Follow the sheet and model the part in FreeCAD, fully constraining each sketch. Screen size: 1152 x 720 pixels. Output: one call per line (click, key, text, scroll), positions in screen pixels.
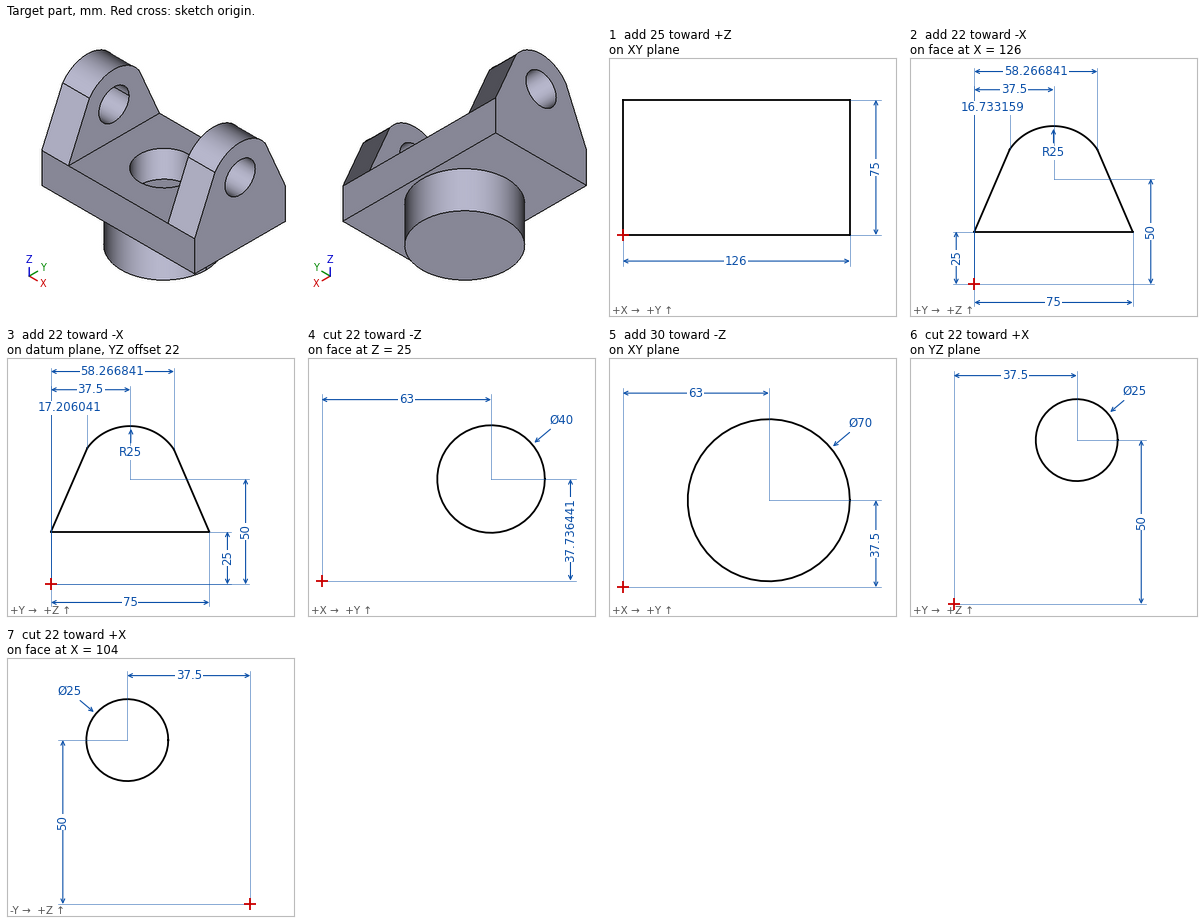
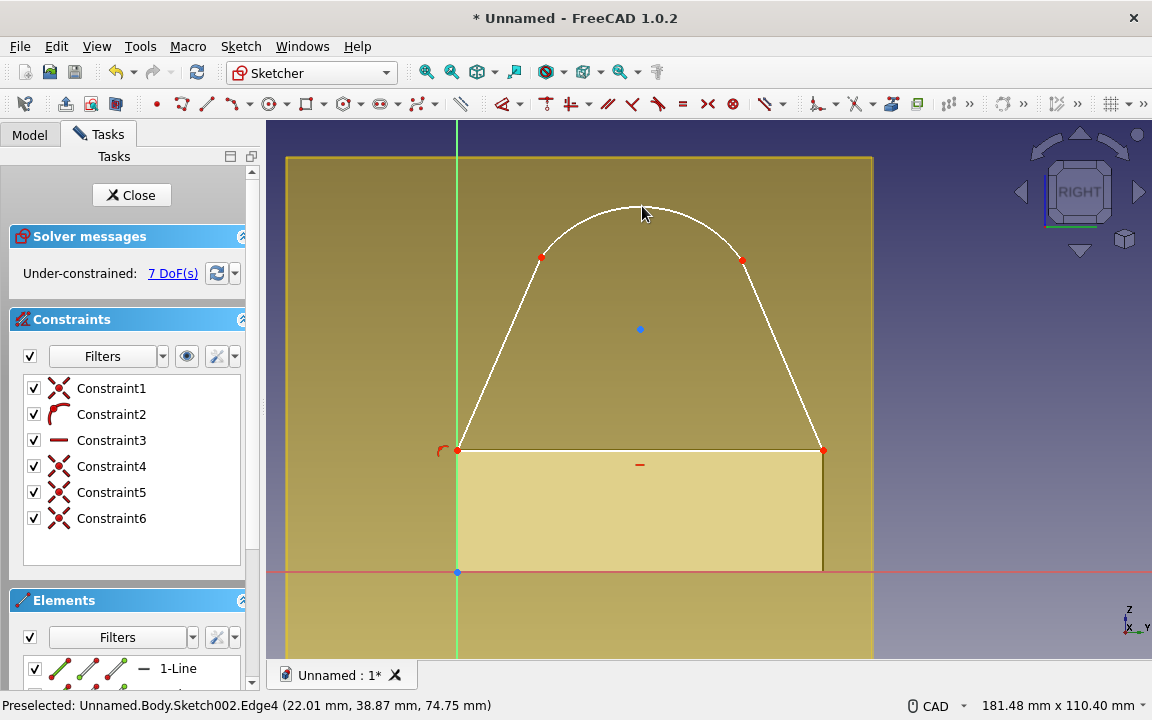
click(502, 104)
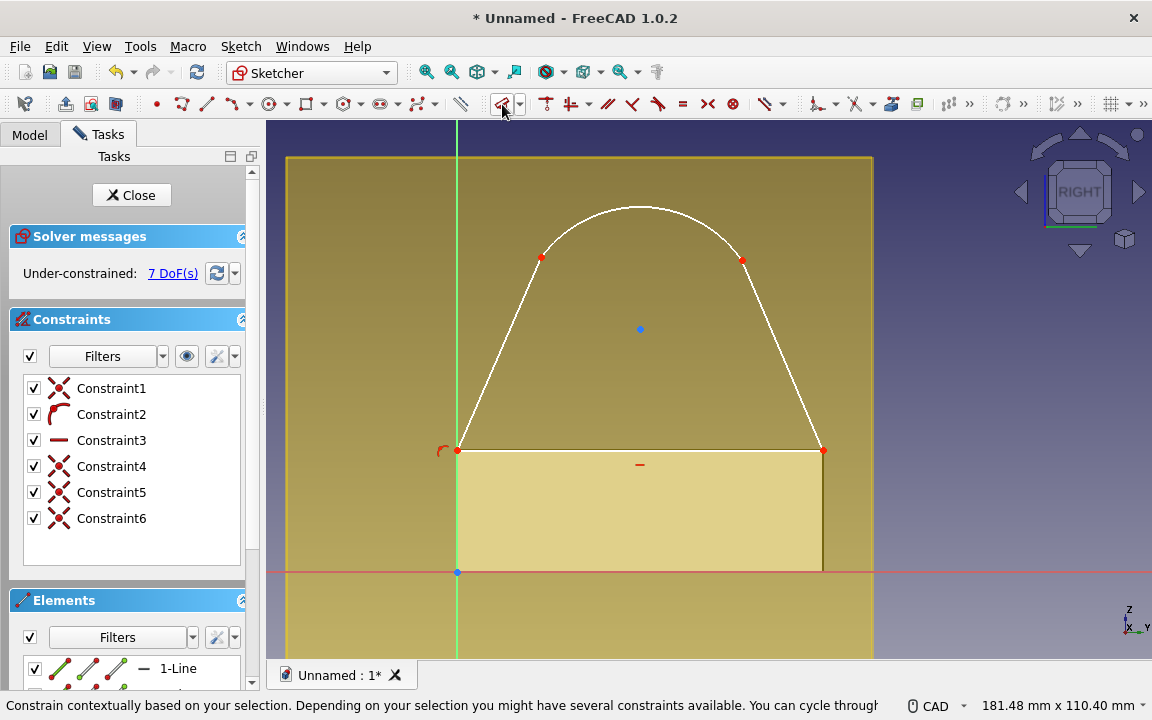
click(688, 217)
click(700, 188)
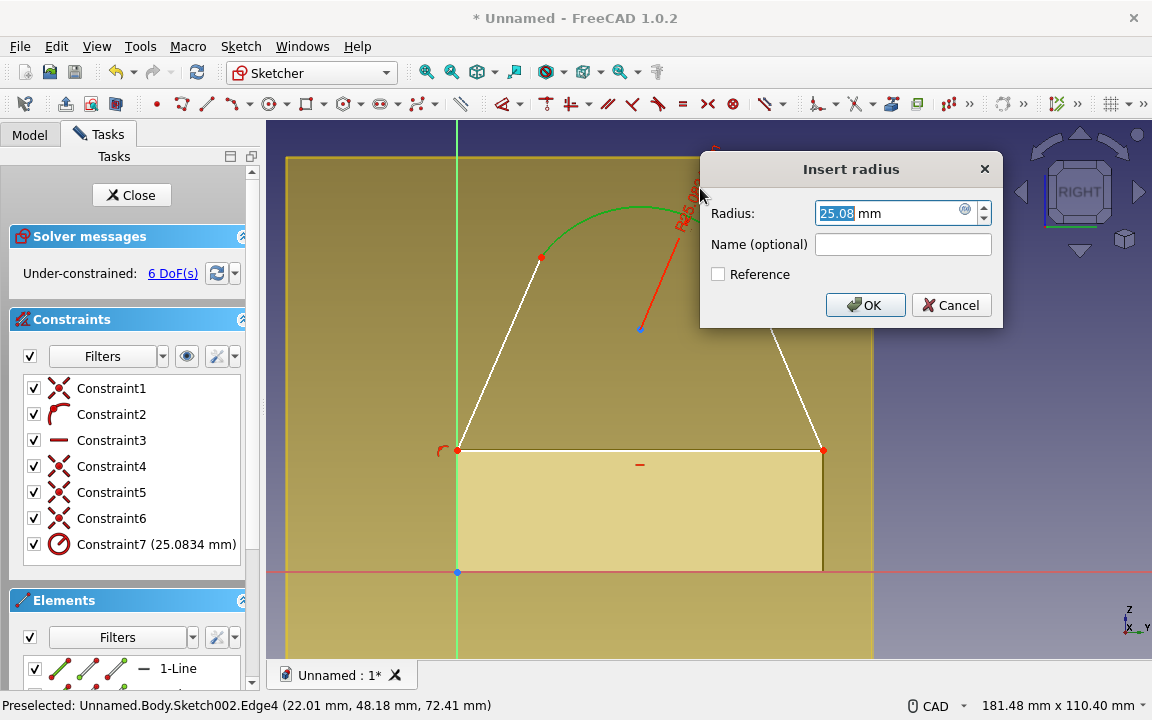
text(25)
key(Return)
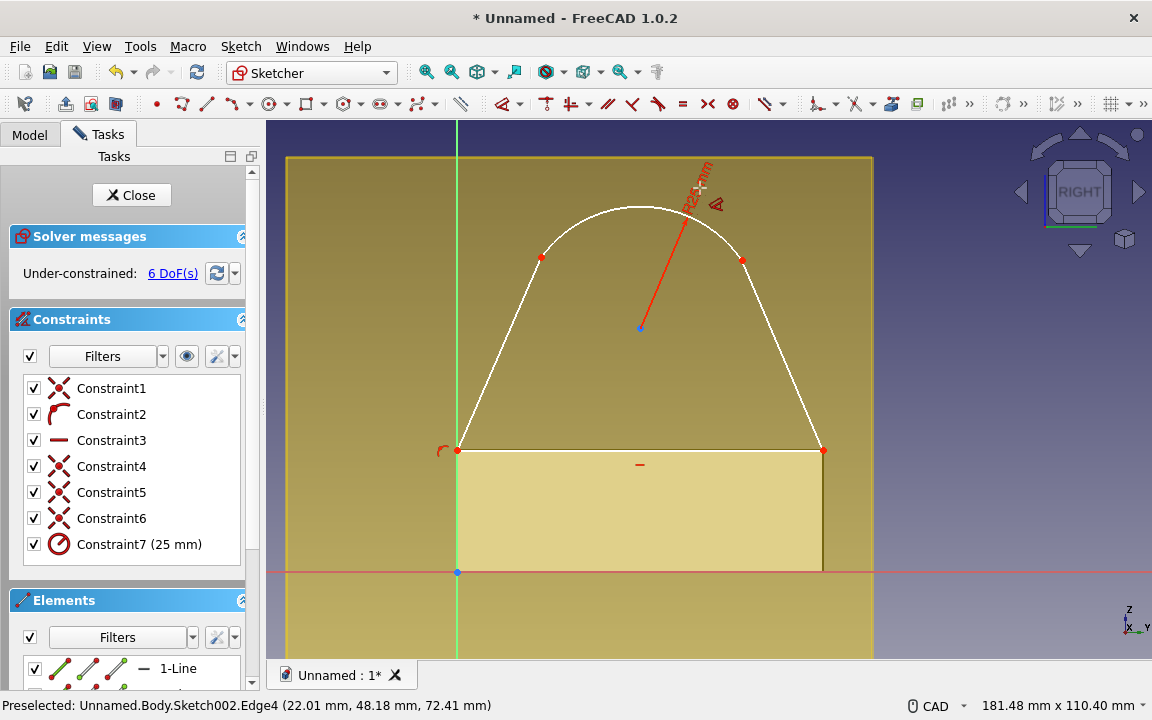
click(713, 451)
click(640, 485)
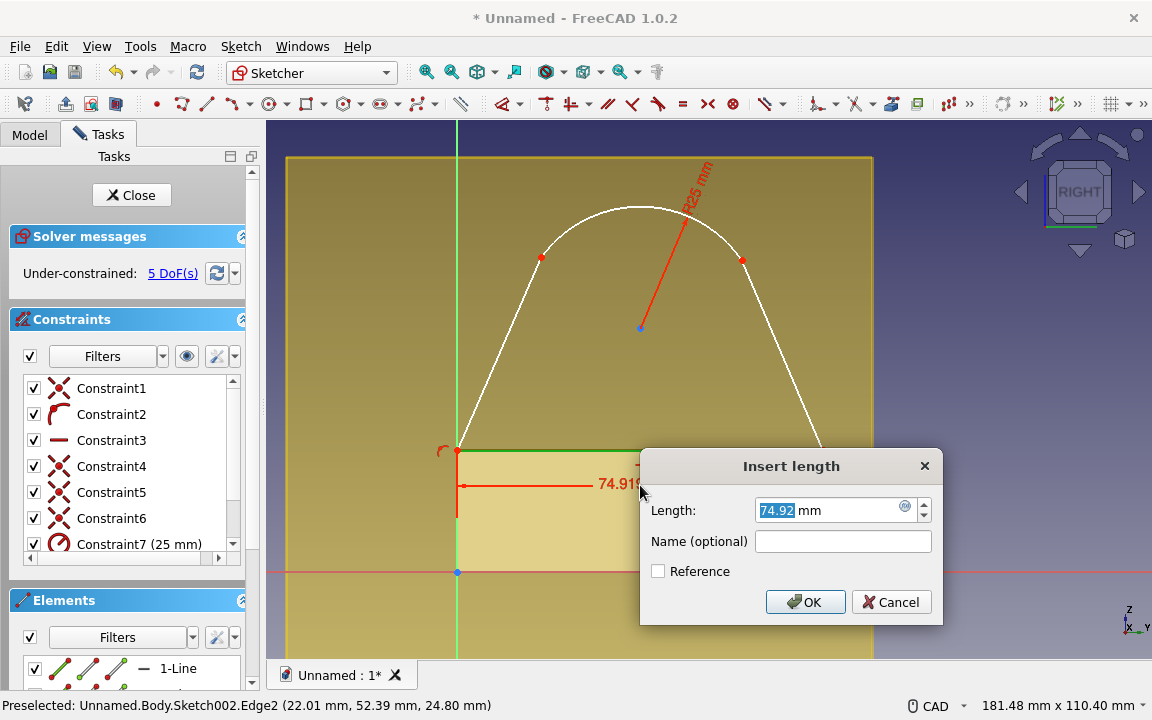
text(75)
key(Return)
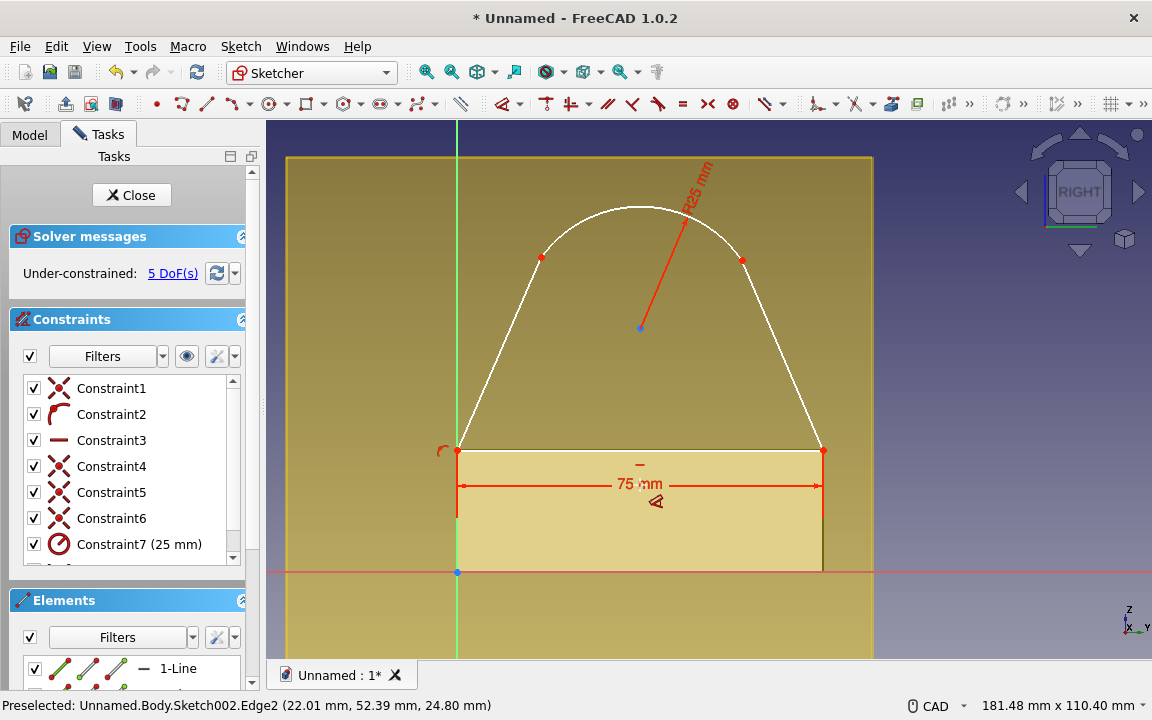
click(823, 451)
click(857, 512)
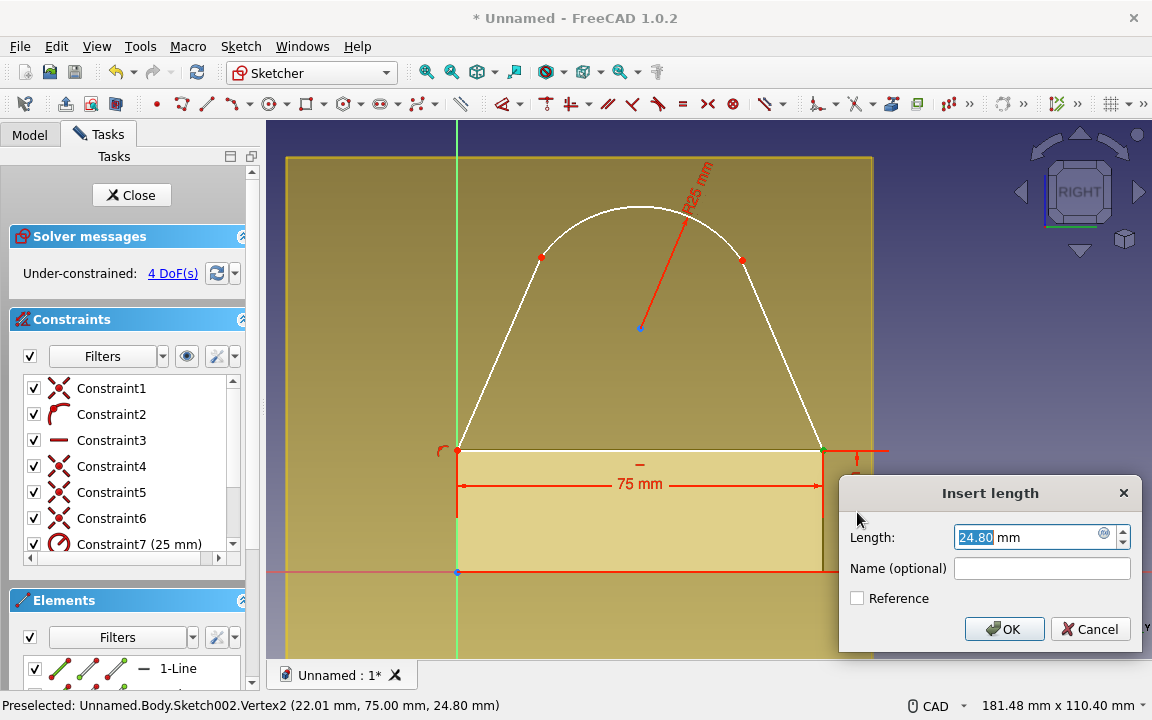
text(25)
key(Return)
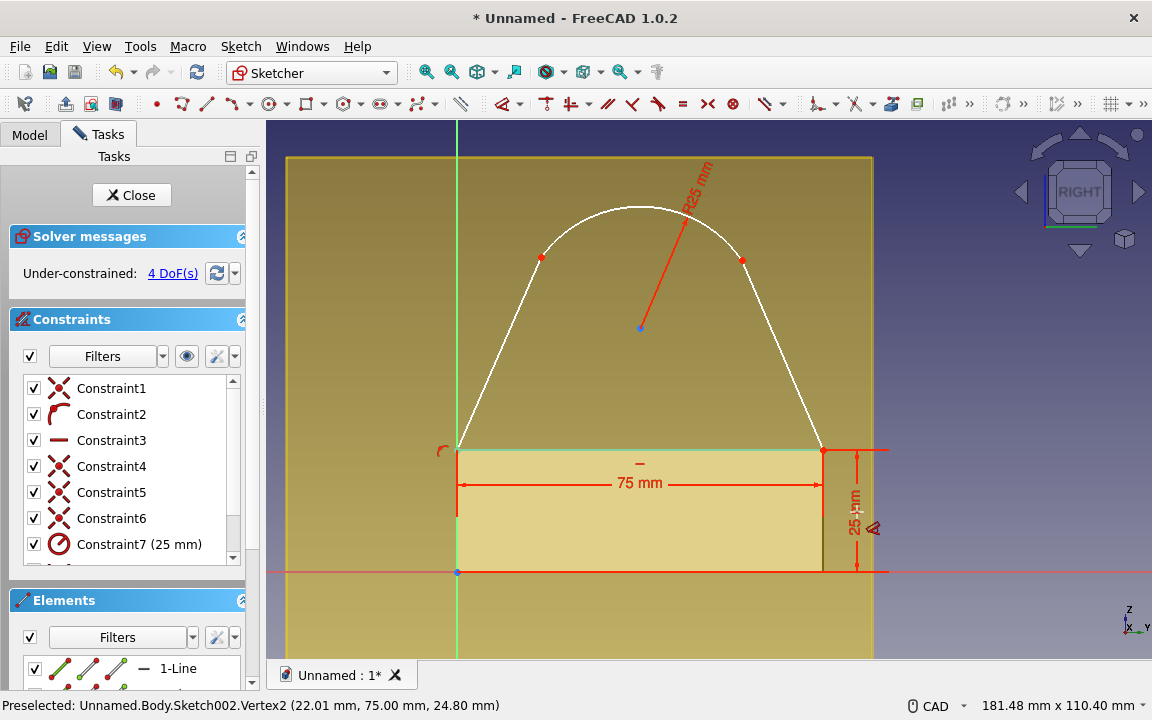
click(640, 329)
click(423, 450)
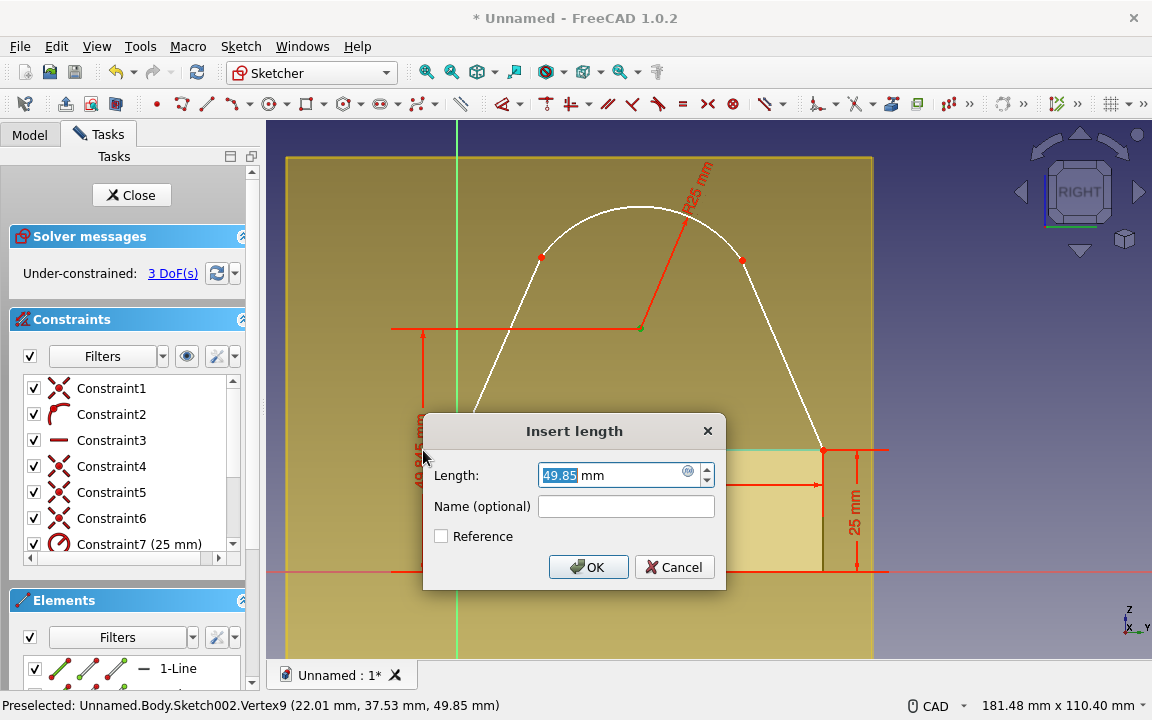
text(50)
key(Return)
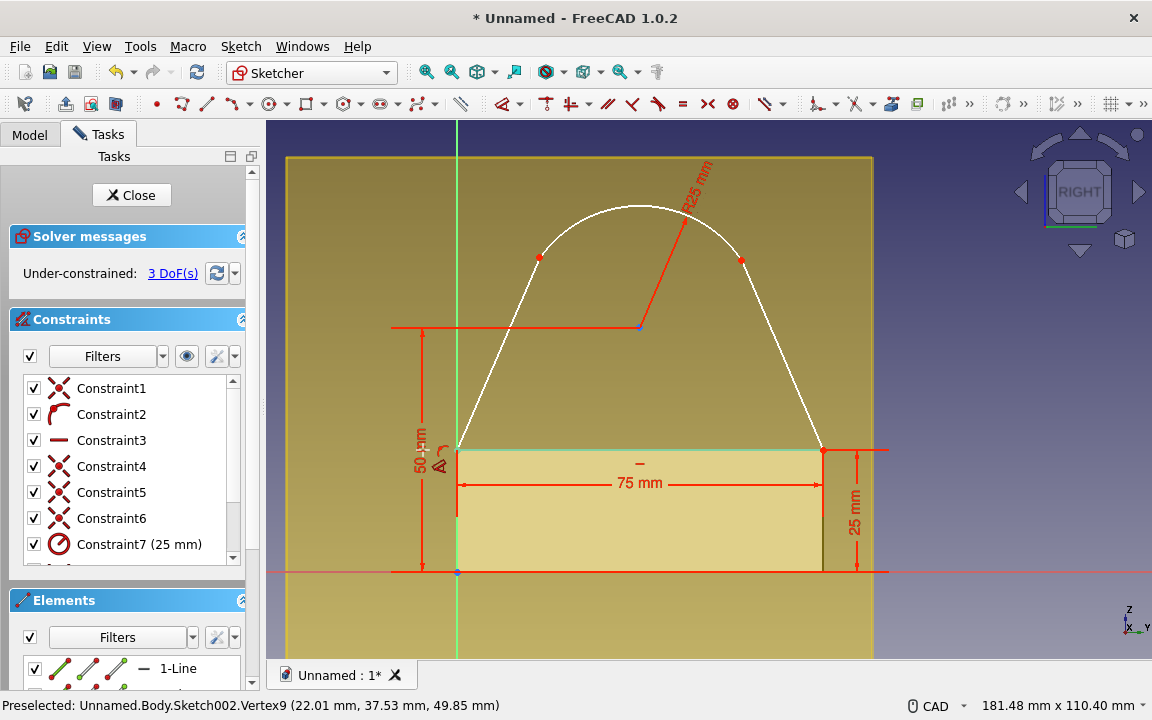
click(640, 328)
click(549, 606)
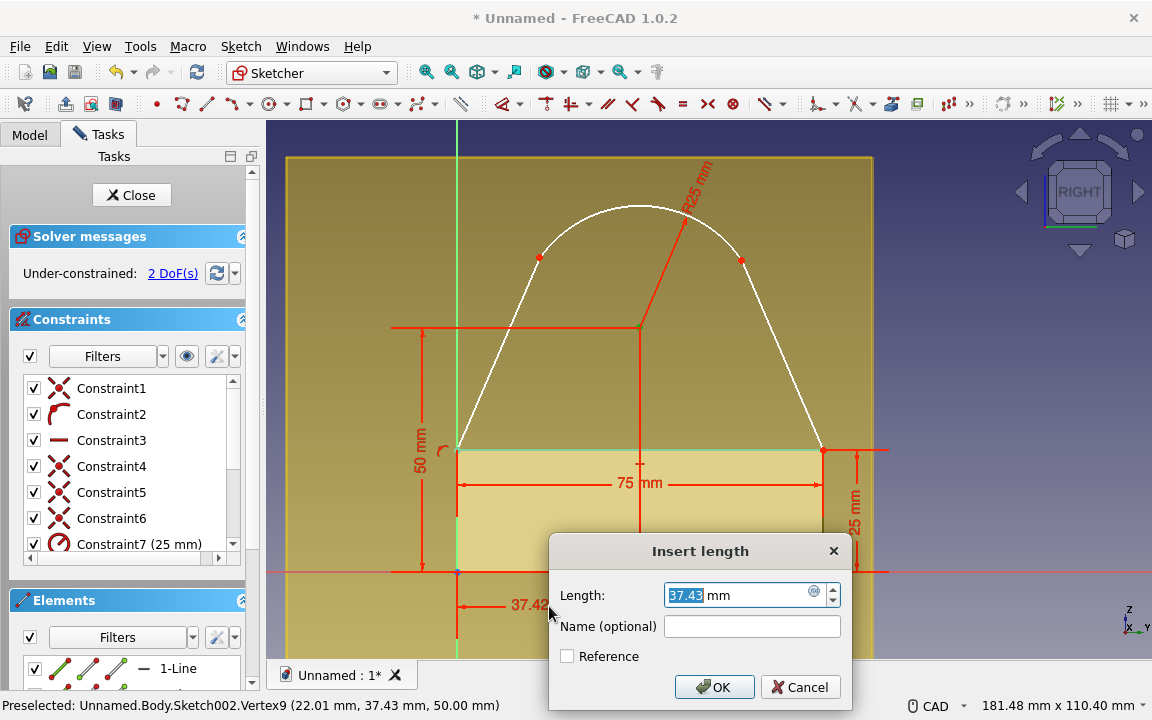
text(37.5)
key(Return)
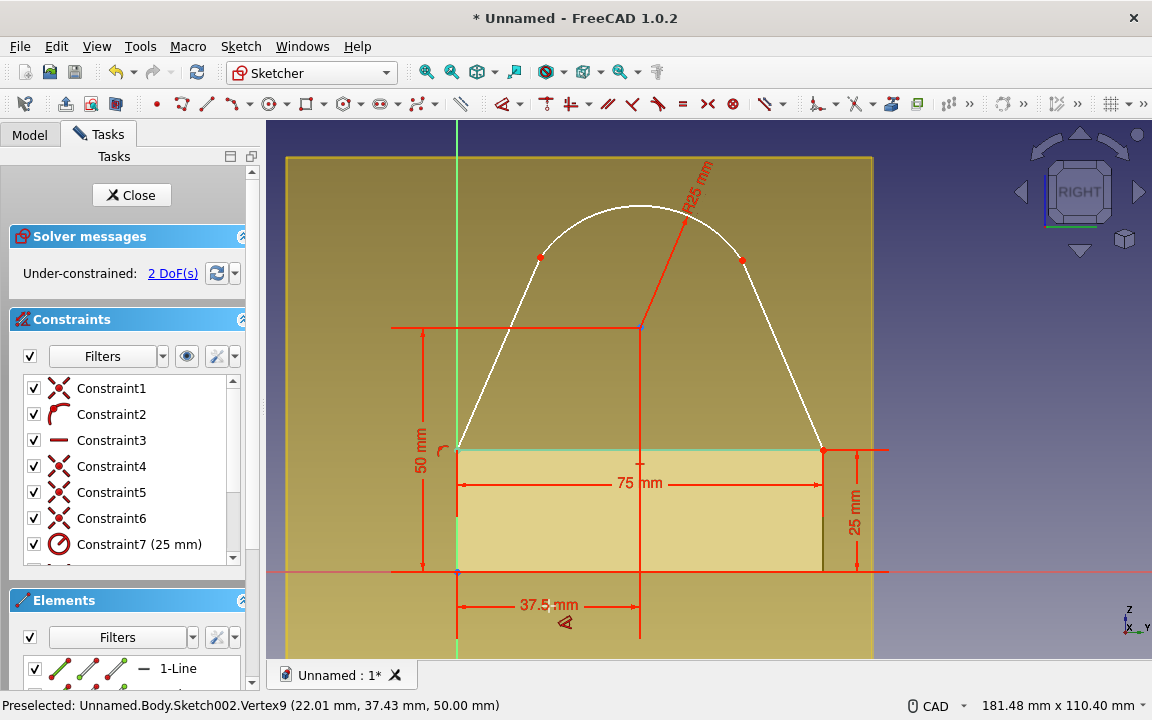
click(742, 261)
click(665, 606)